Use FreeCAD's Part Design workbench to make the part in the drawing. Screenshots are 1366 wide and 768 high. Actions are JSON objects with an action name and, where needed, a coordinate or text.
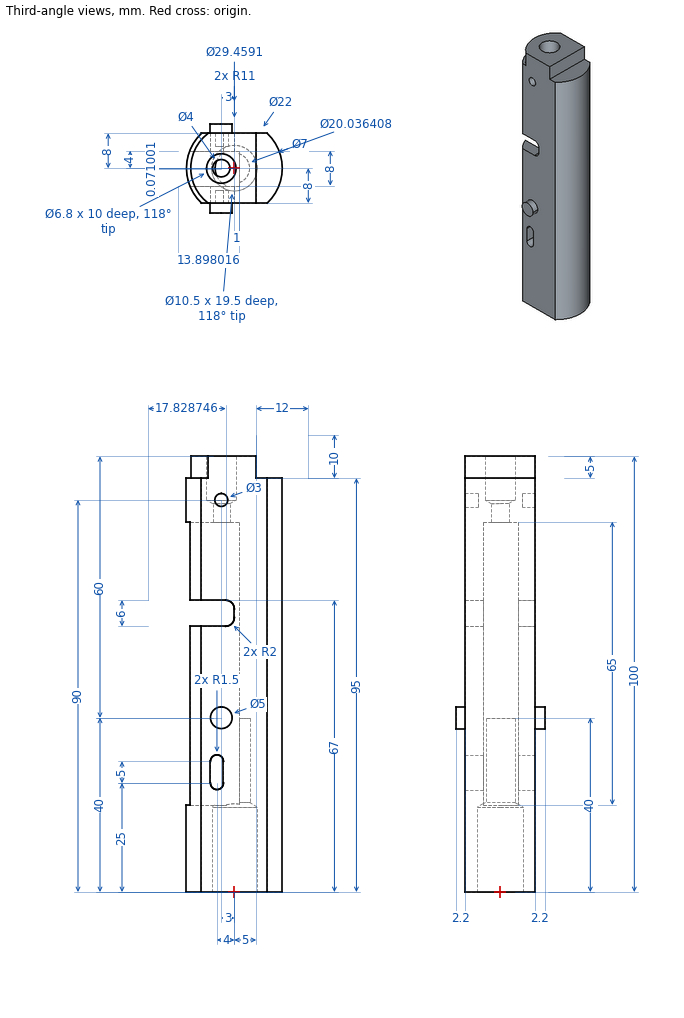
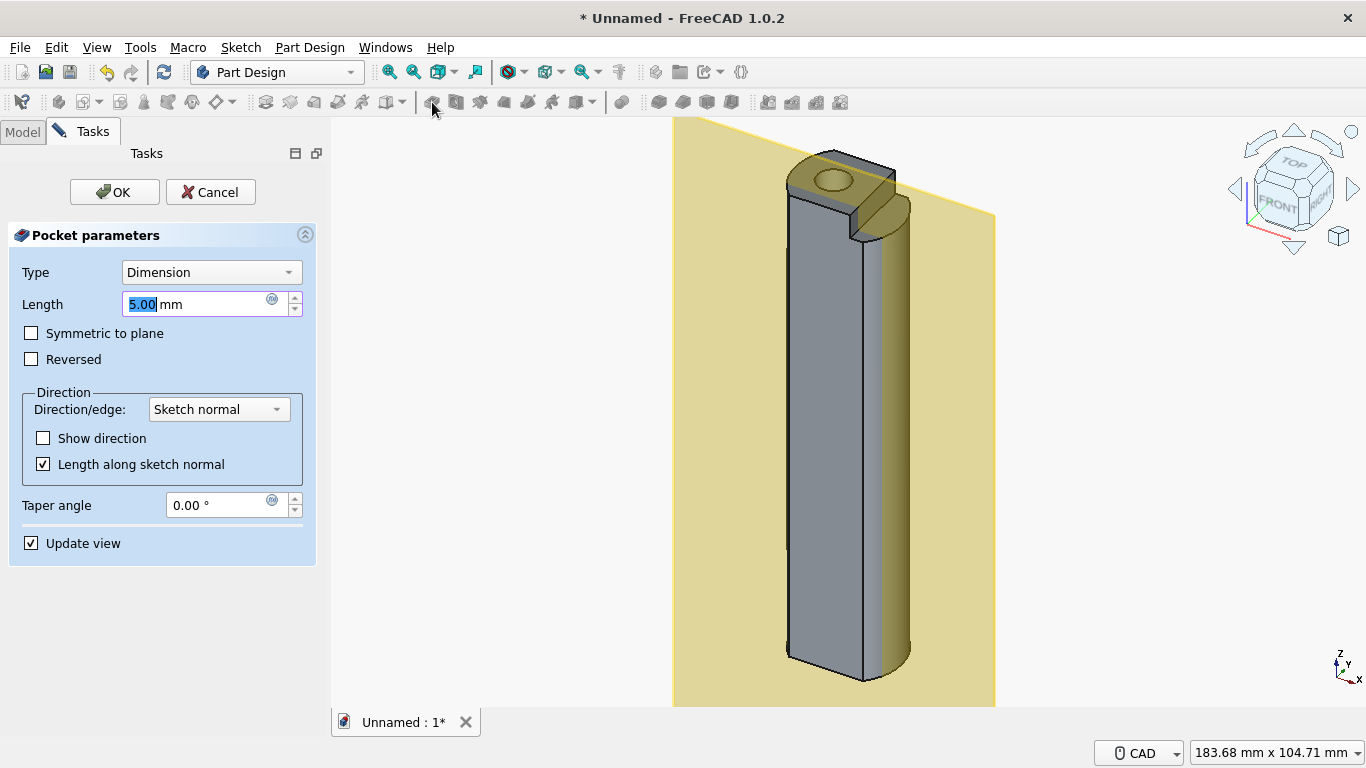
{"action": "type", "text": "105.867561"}
{"action": "key", "text": "Tab"}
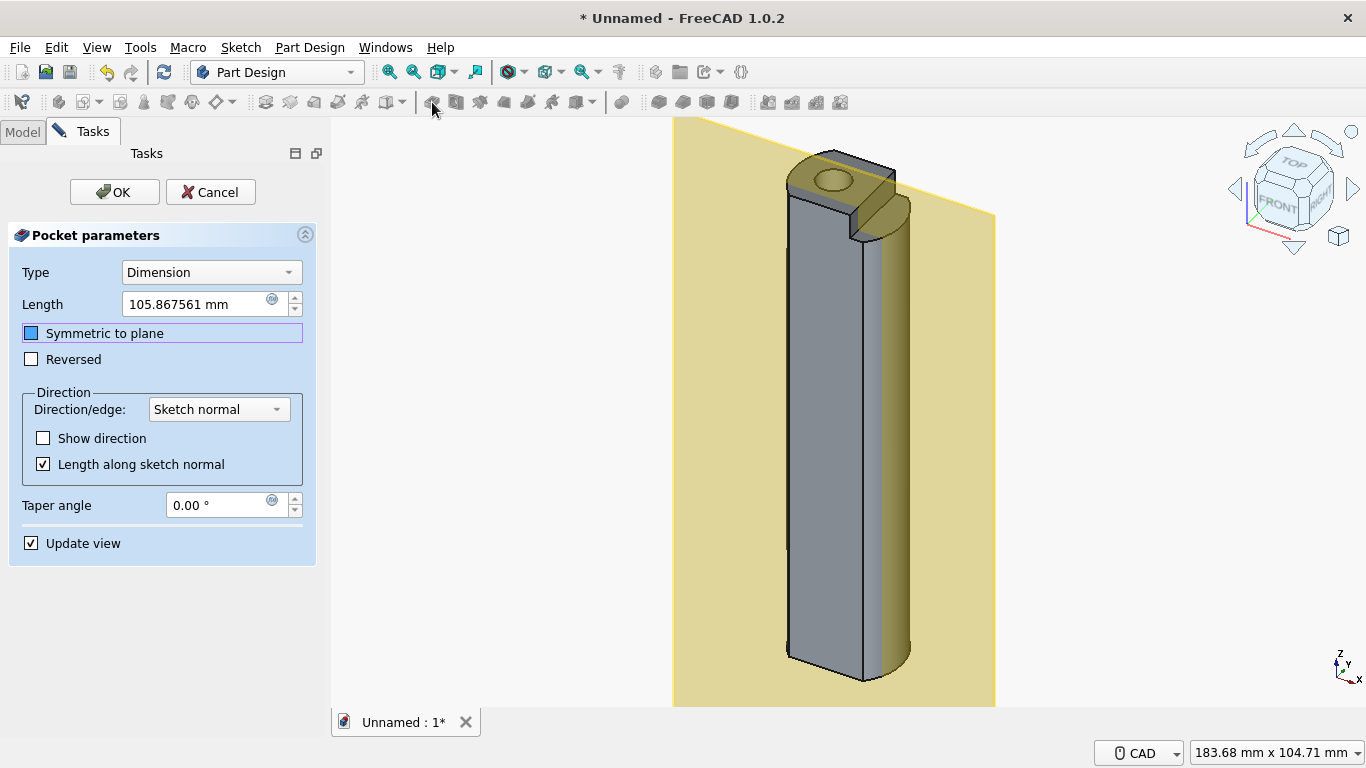
{"action": "left_click", "coordinate": [30, 359]}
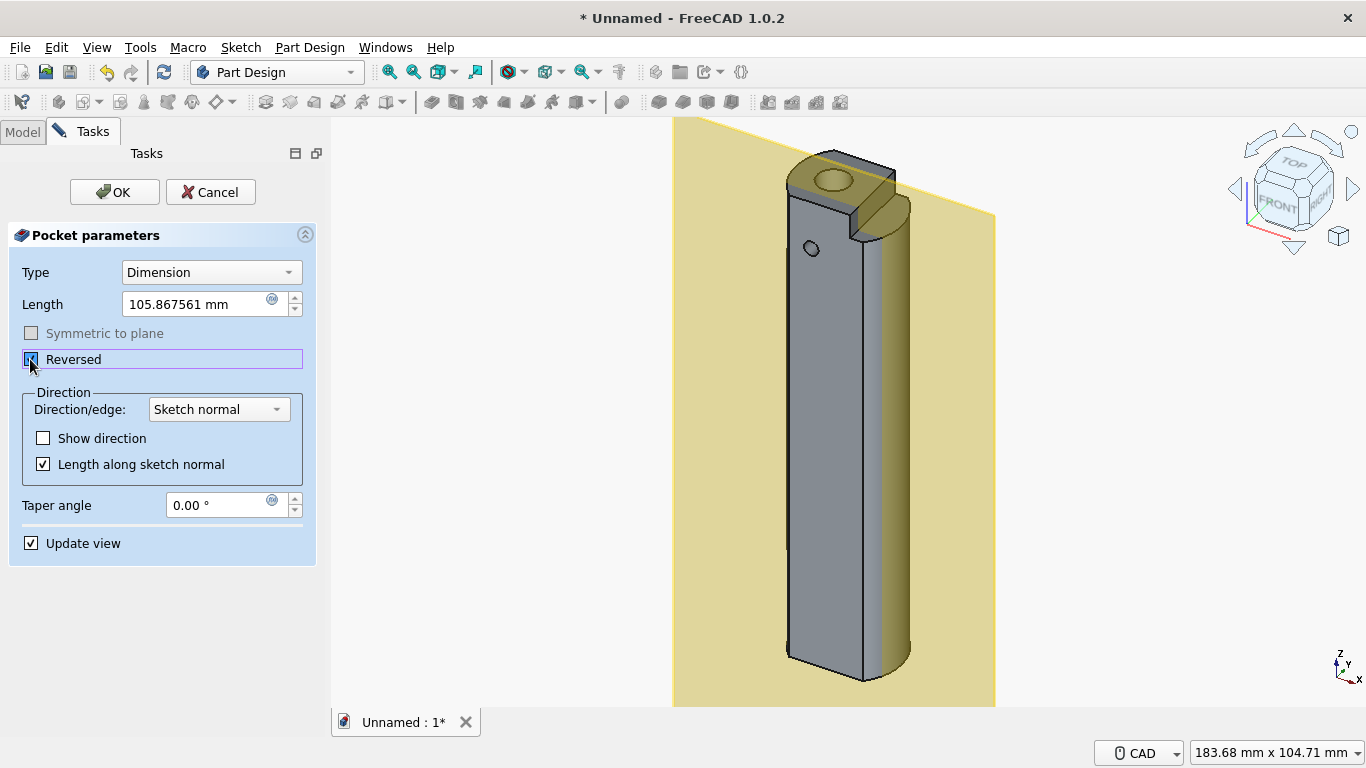
{"action": "left_click", "coordinate": [115, 192]}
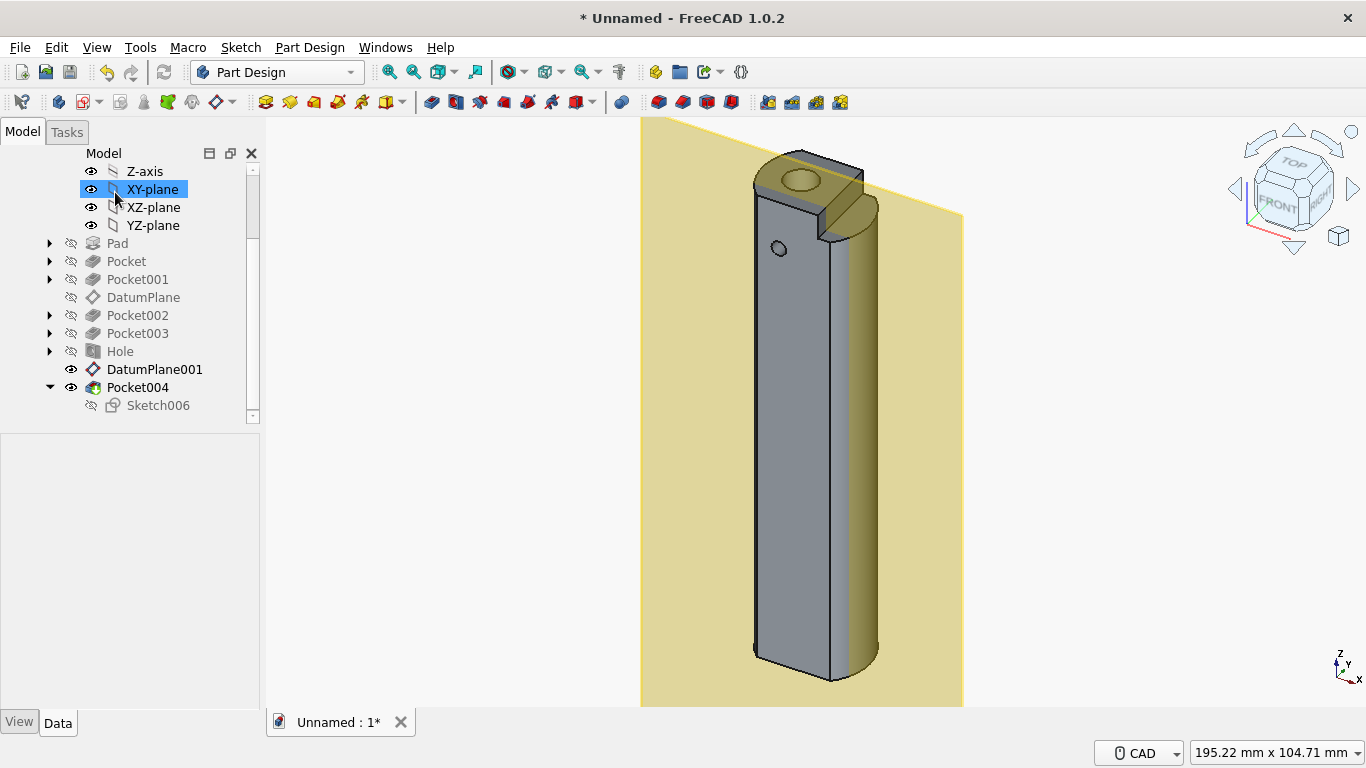
{"action": "left_click", "coordinate": [116, 369]}
{"action": "key", "text": "space"}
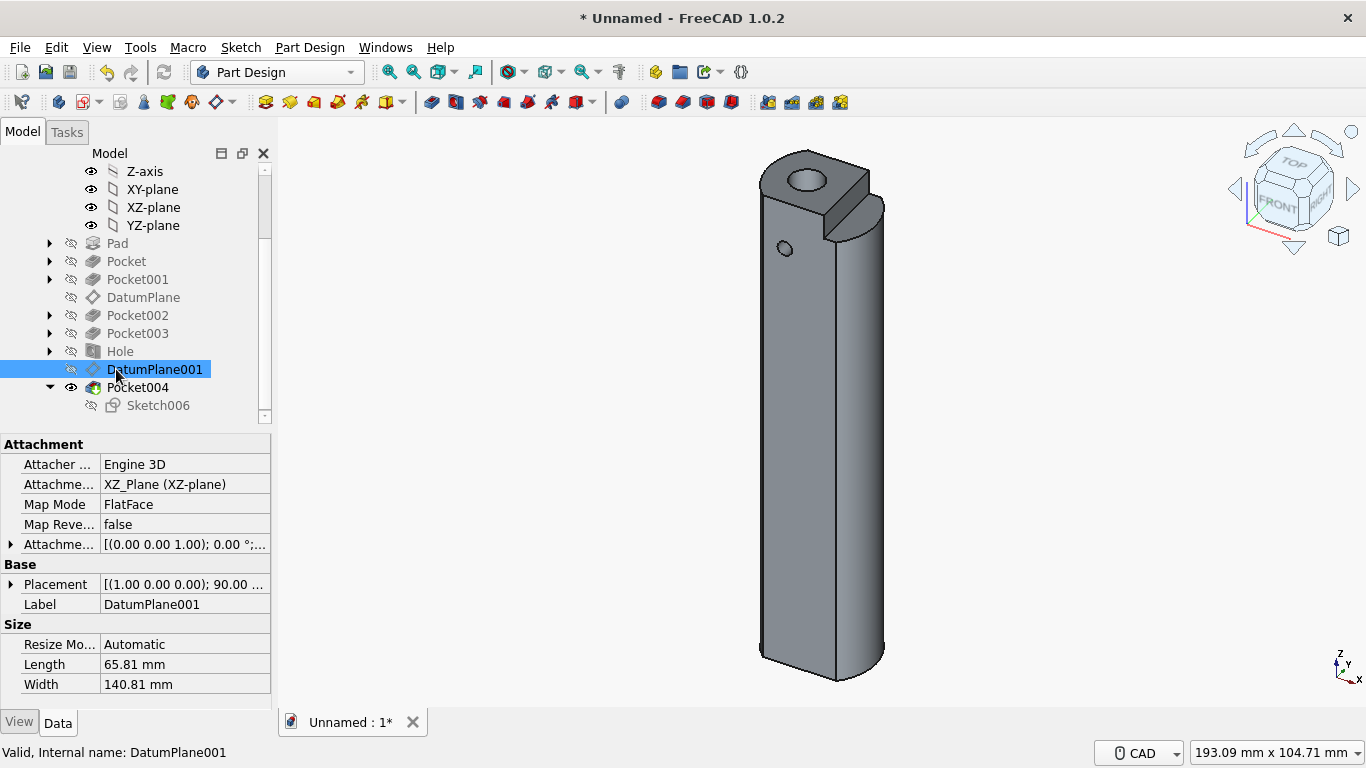
{"action": "left_click", "coordinate": [116, 387]}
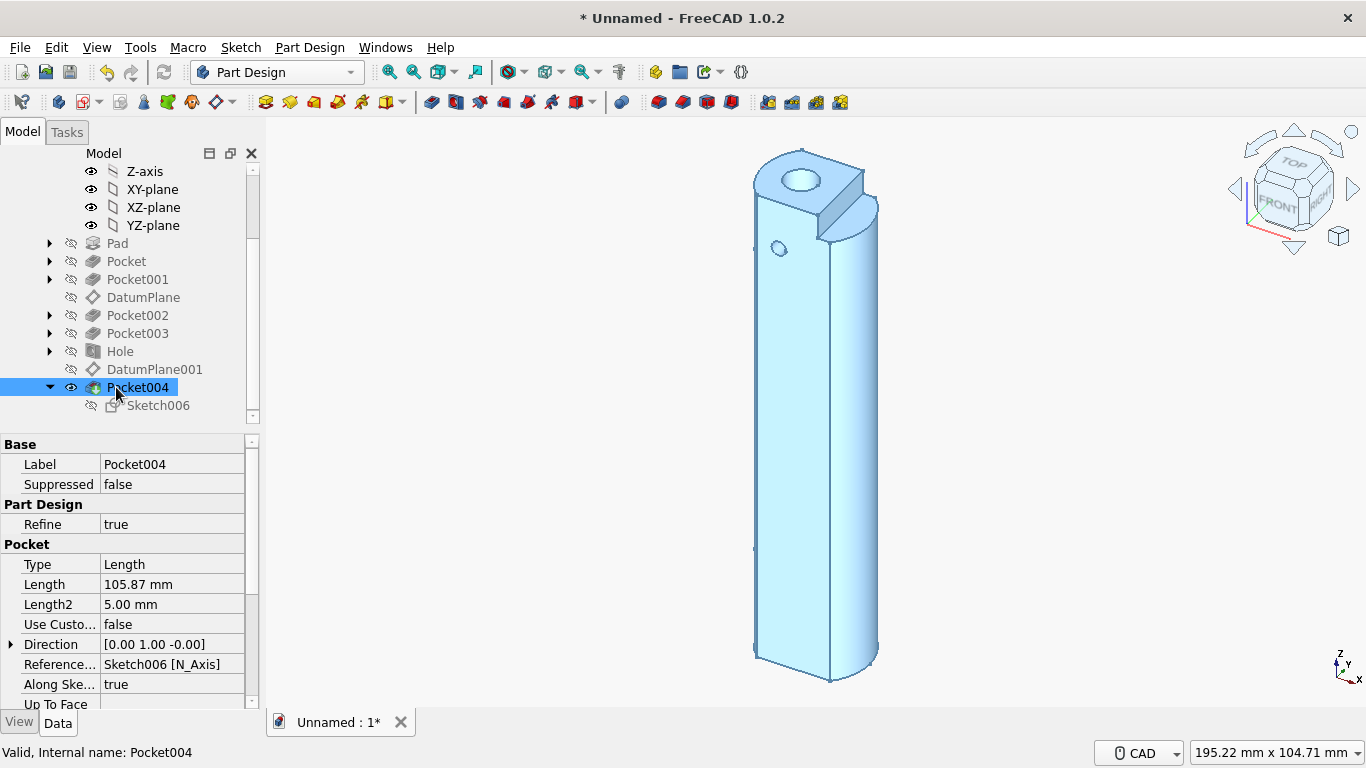
{"action": "left_click", "coordinate": [768, 102]}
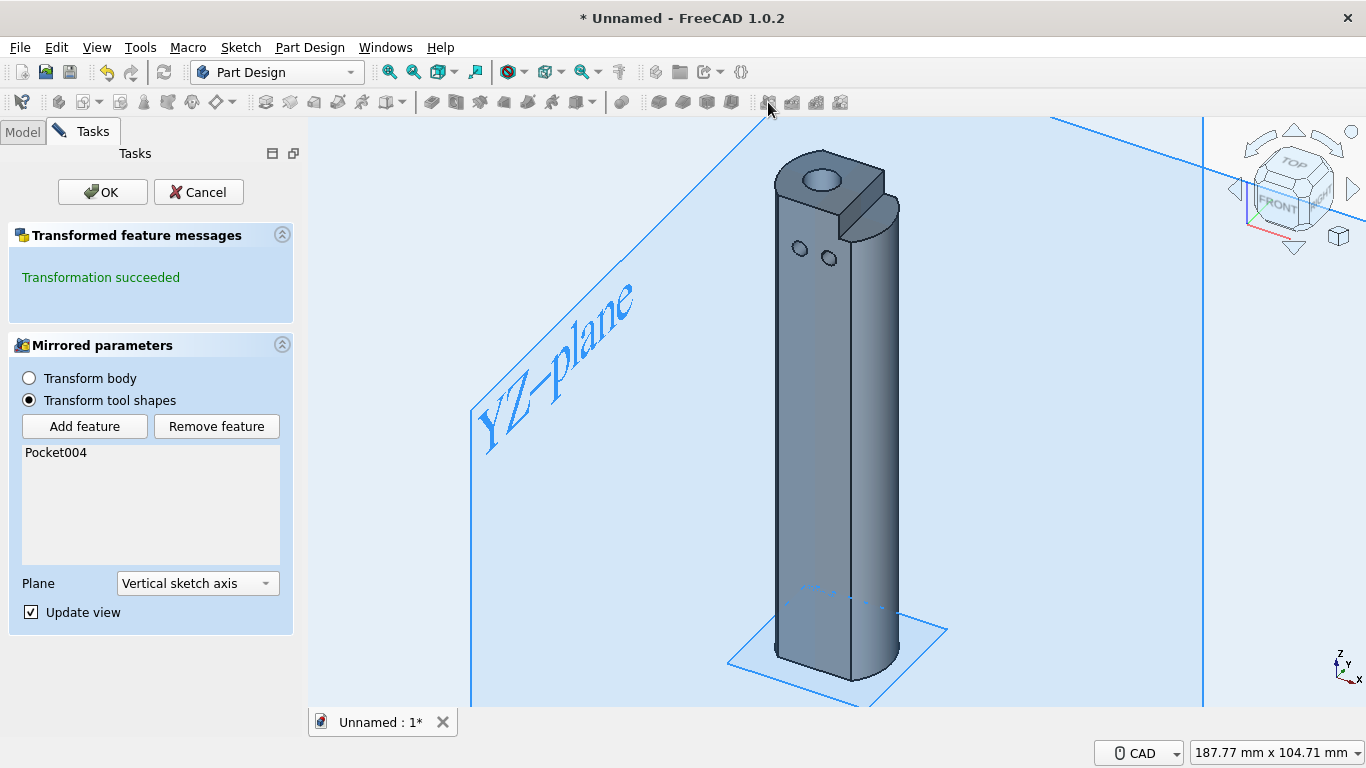
{"action": "left_click", "coordinate": [198, 584]}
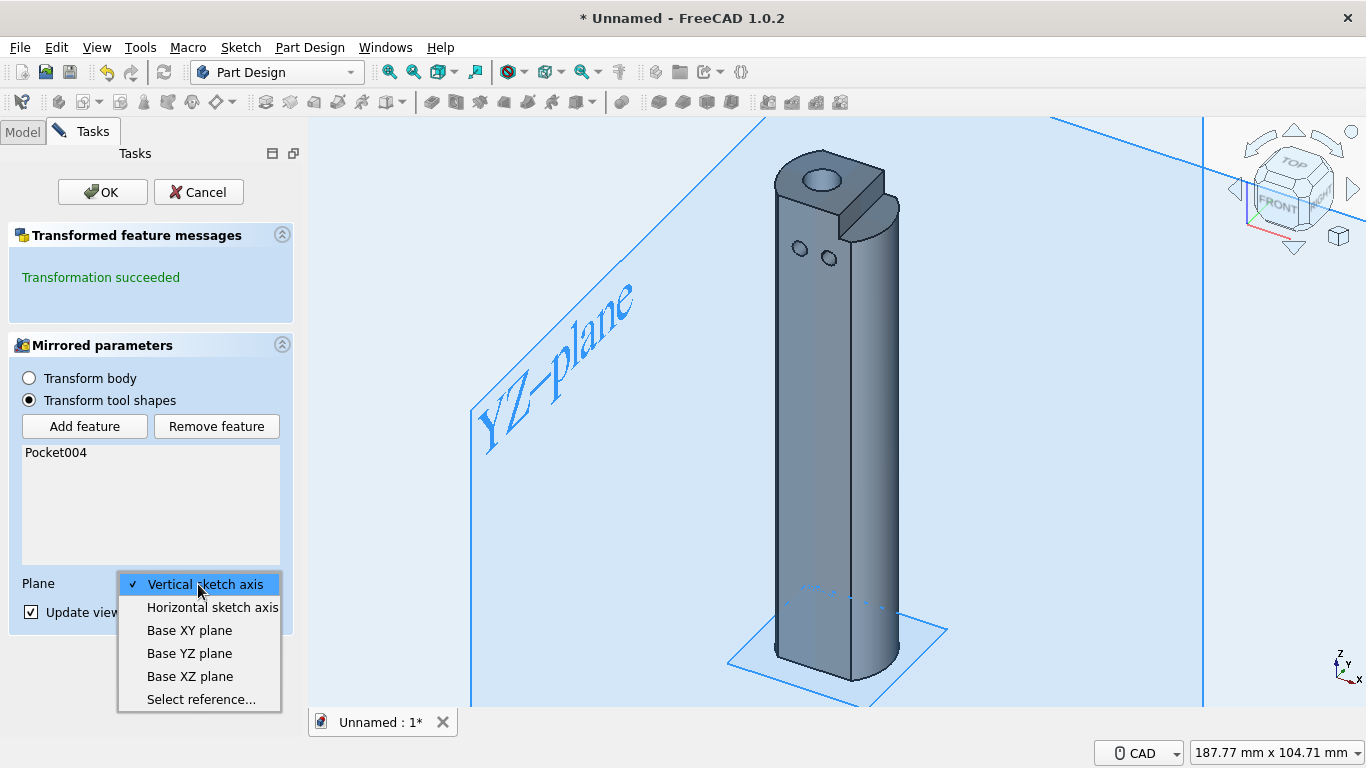
{"action": "left_click", "coordinate": [198, 676]}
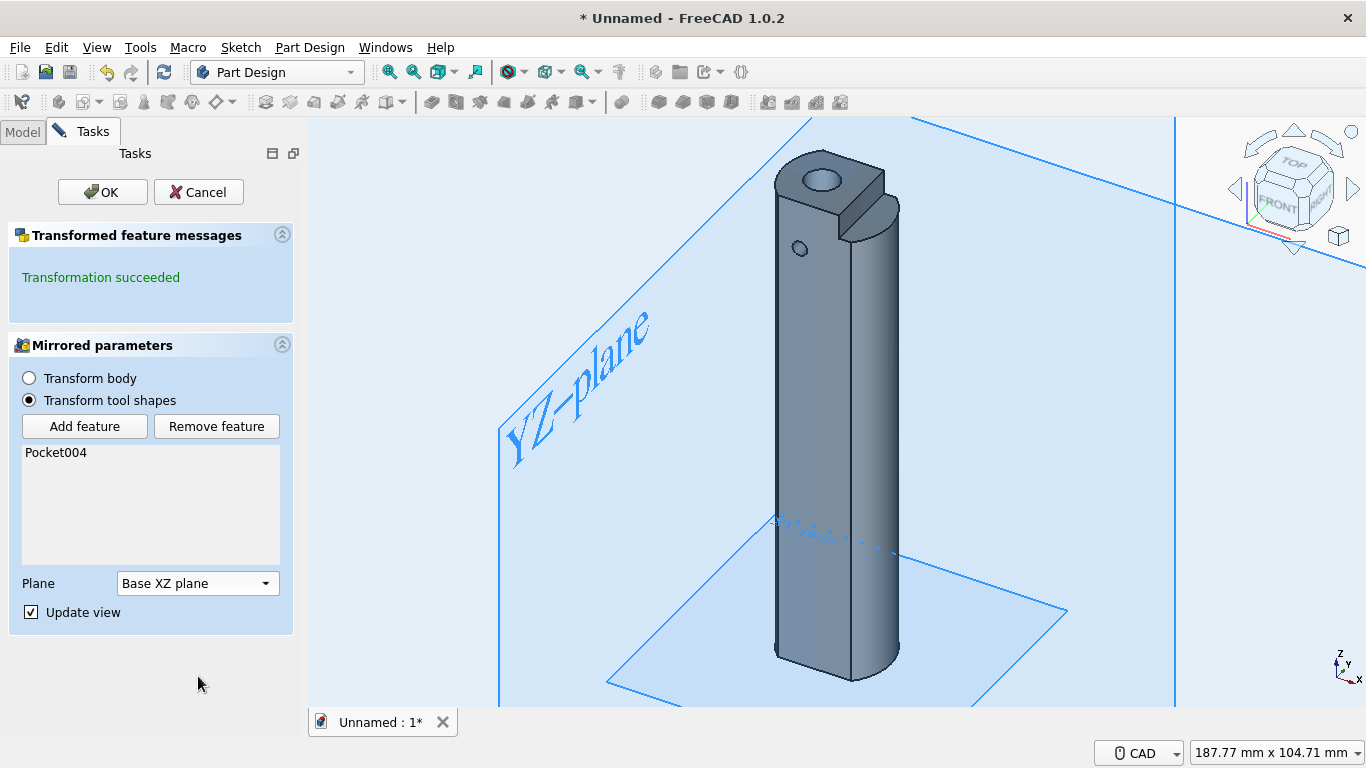
{"action": "left_click", "coordinate": [103, 192]}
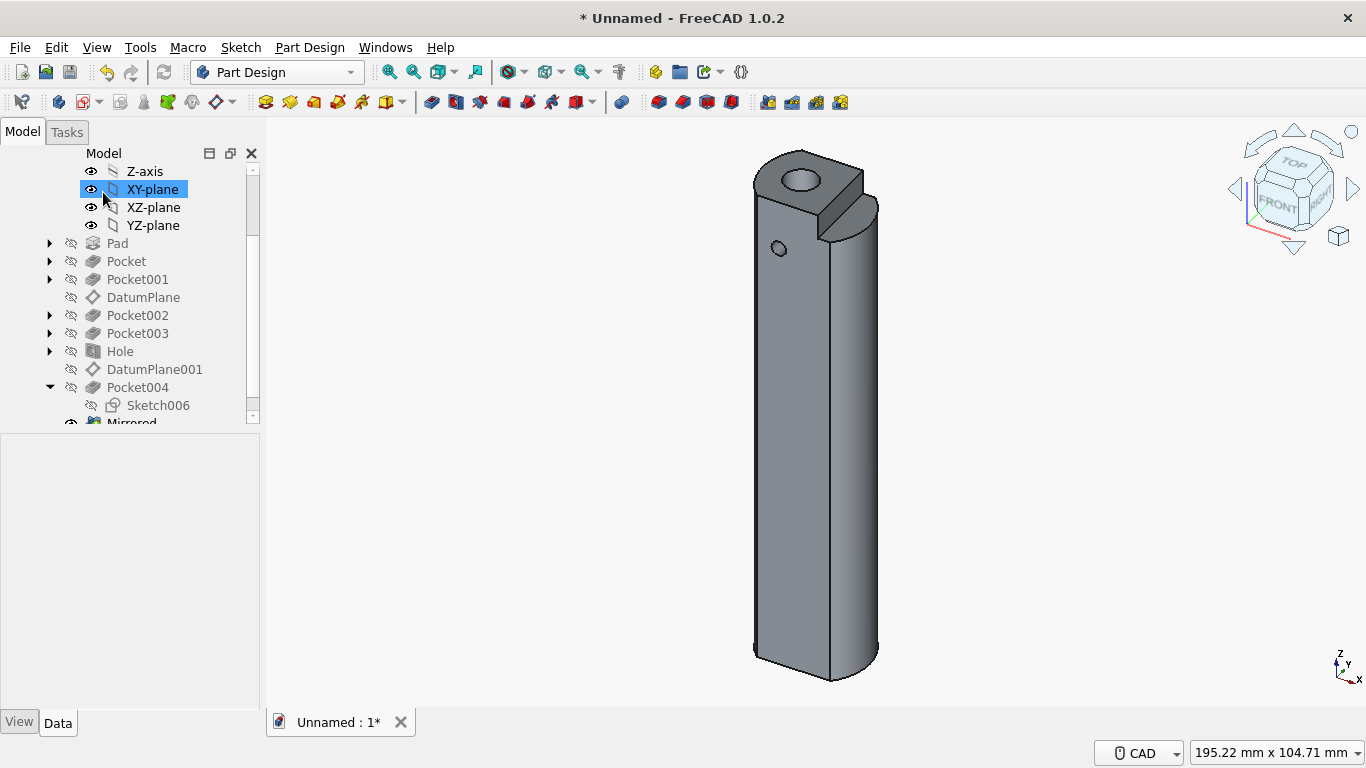
{"action": "left_click", "coordinate": [793, 305]}